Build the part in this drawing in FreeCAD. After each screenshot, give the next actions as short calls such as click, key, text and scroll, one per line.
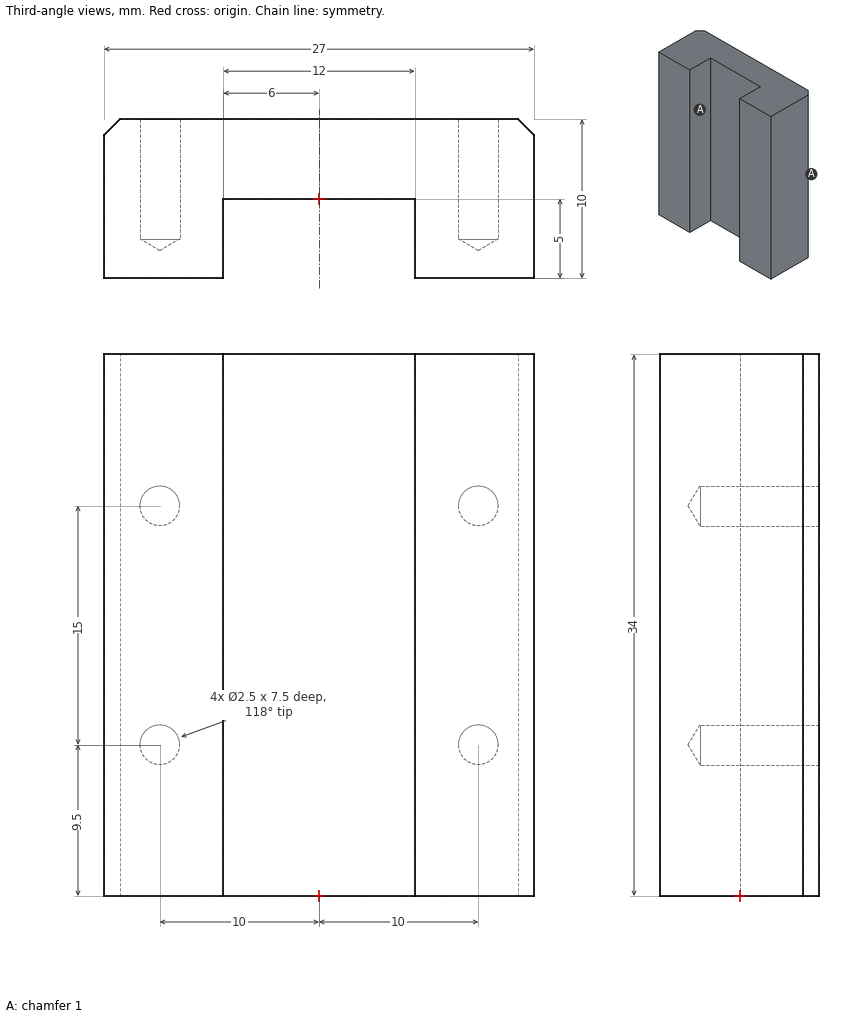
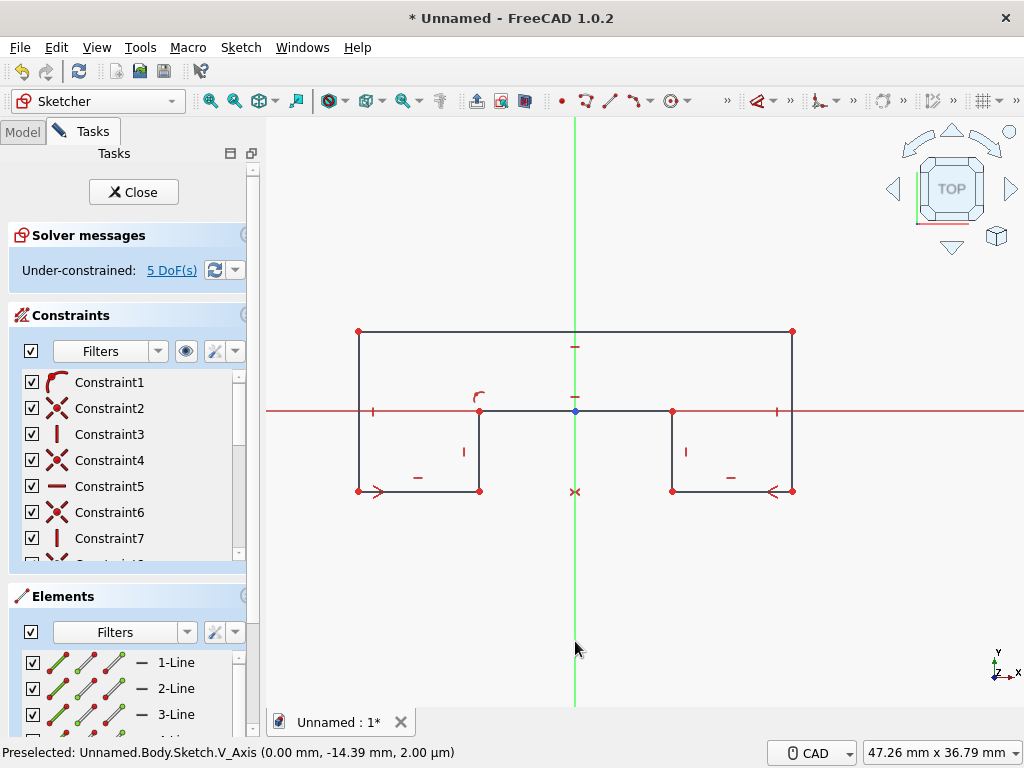
key(d)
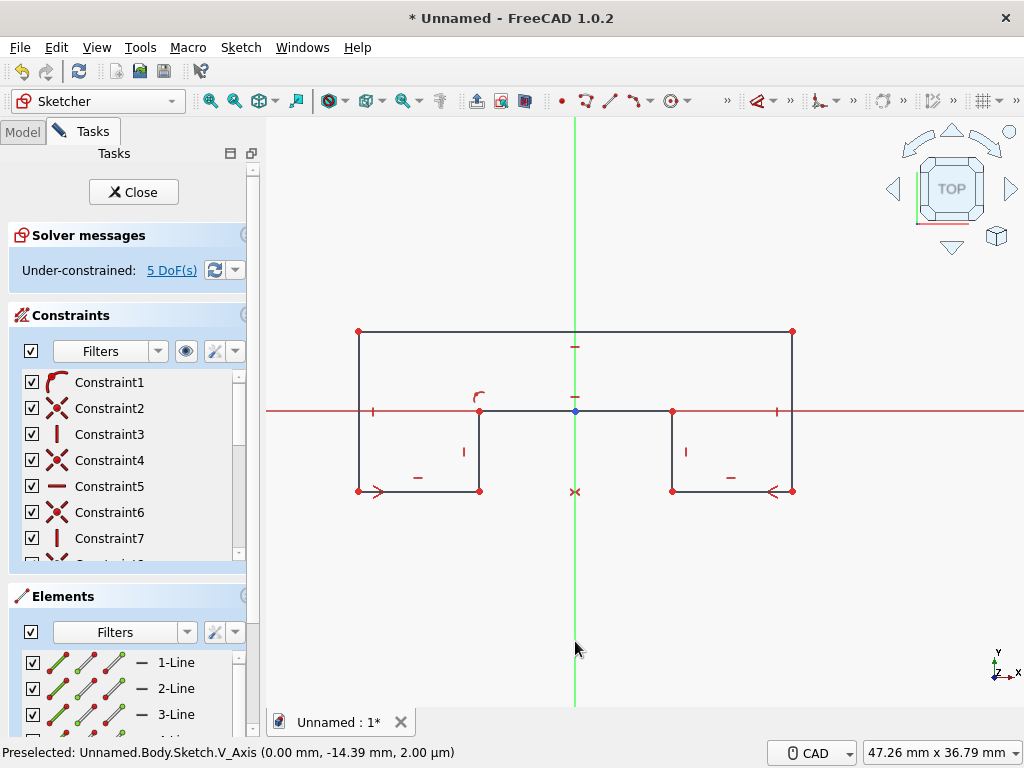
click(672, 435)
click(706, 452)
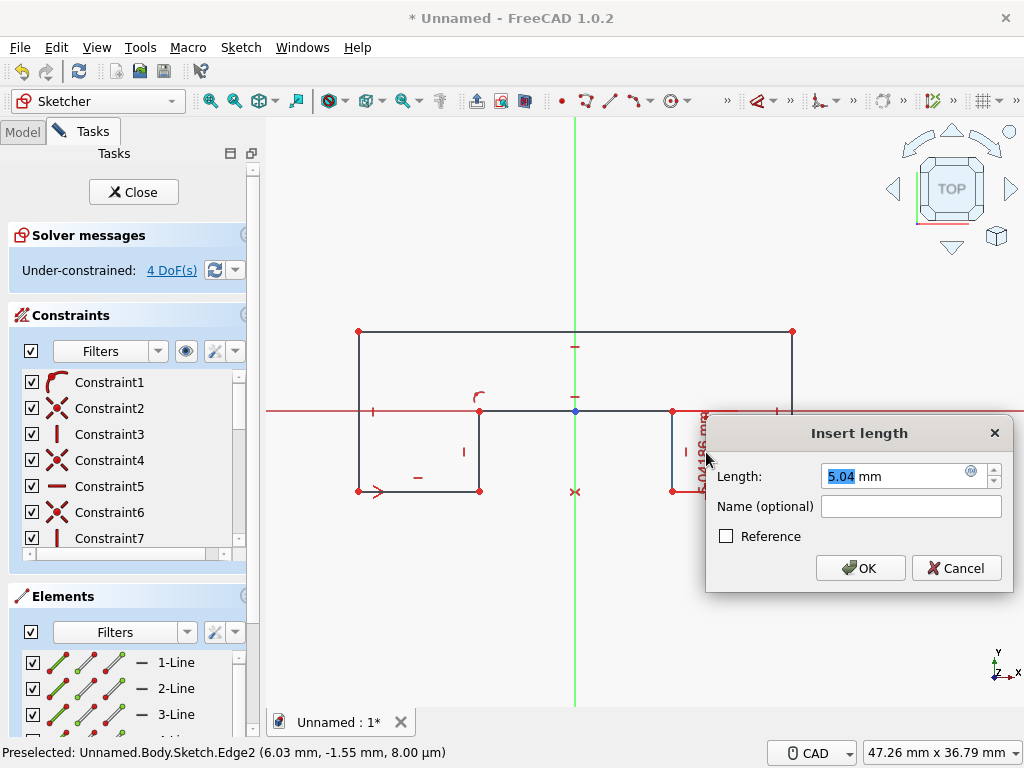
text(5)
key(Return)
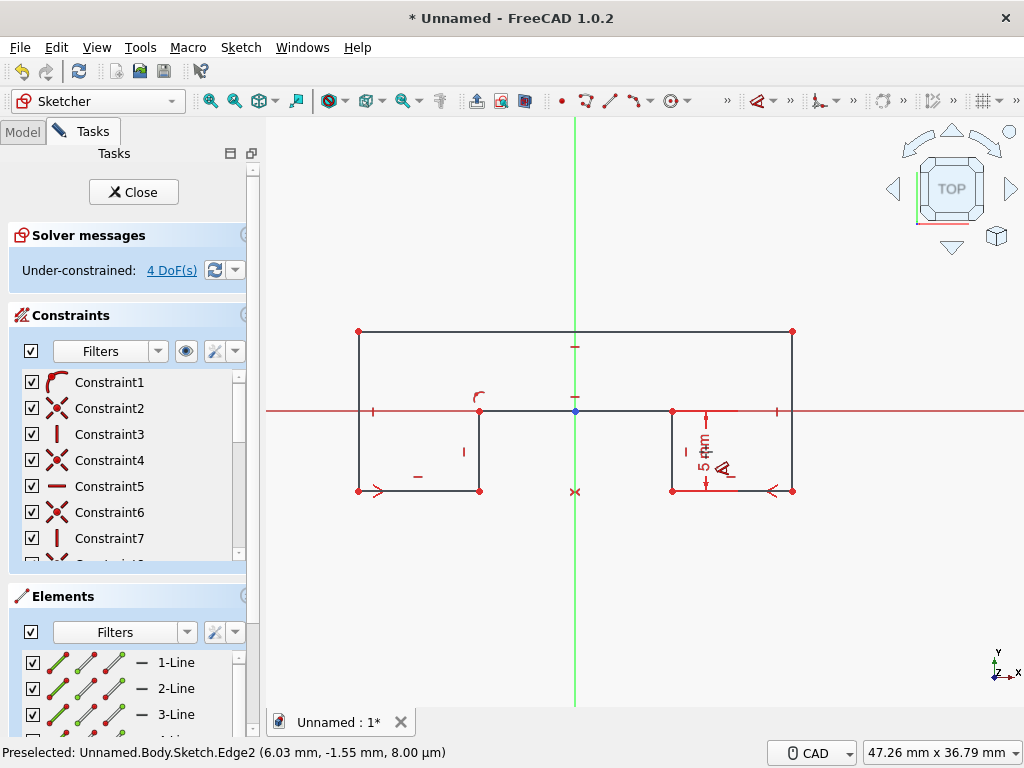
click(537, 411)
click(531, 445)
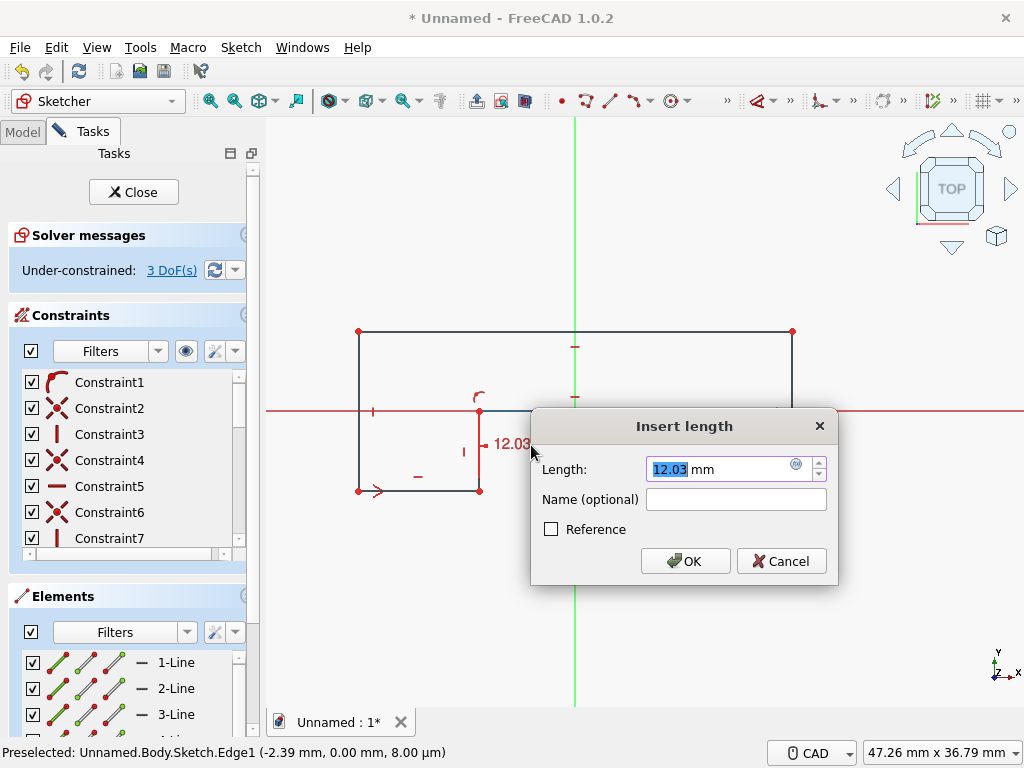
text(12)
key(Return)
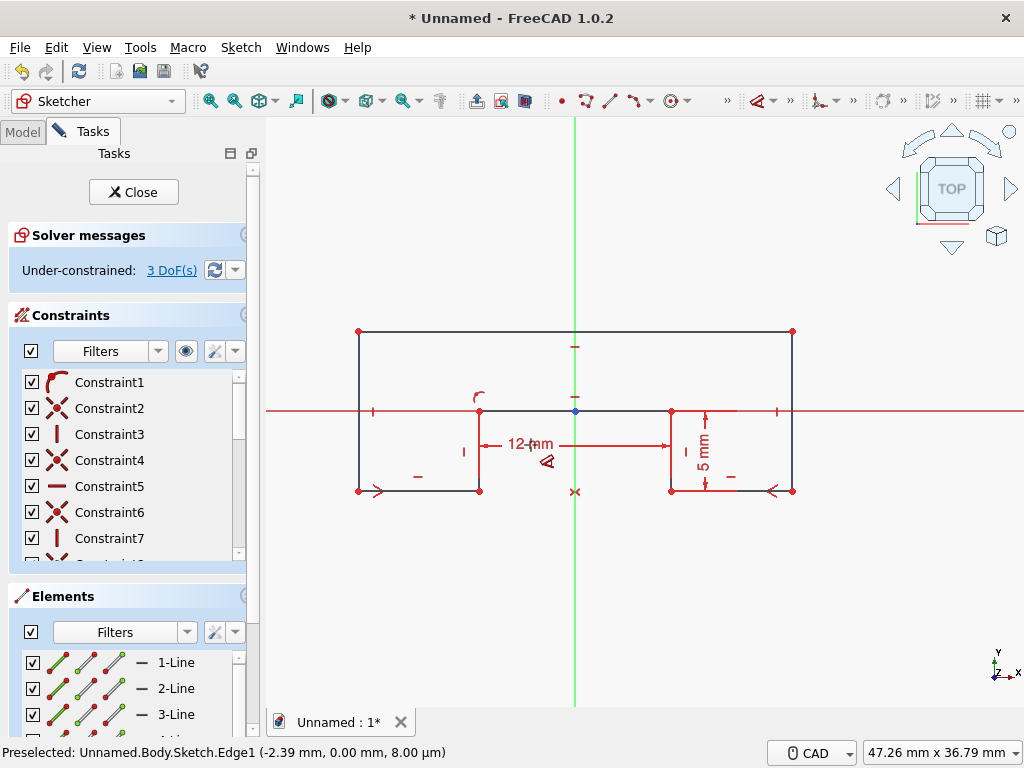
click(792, 444)
click(826, 375)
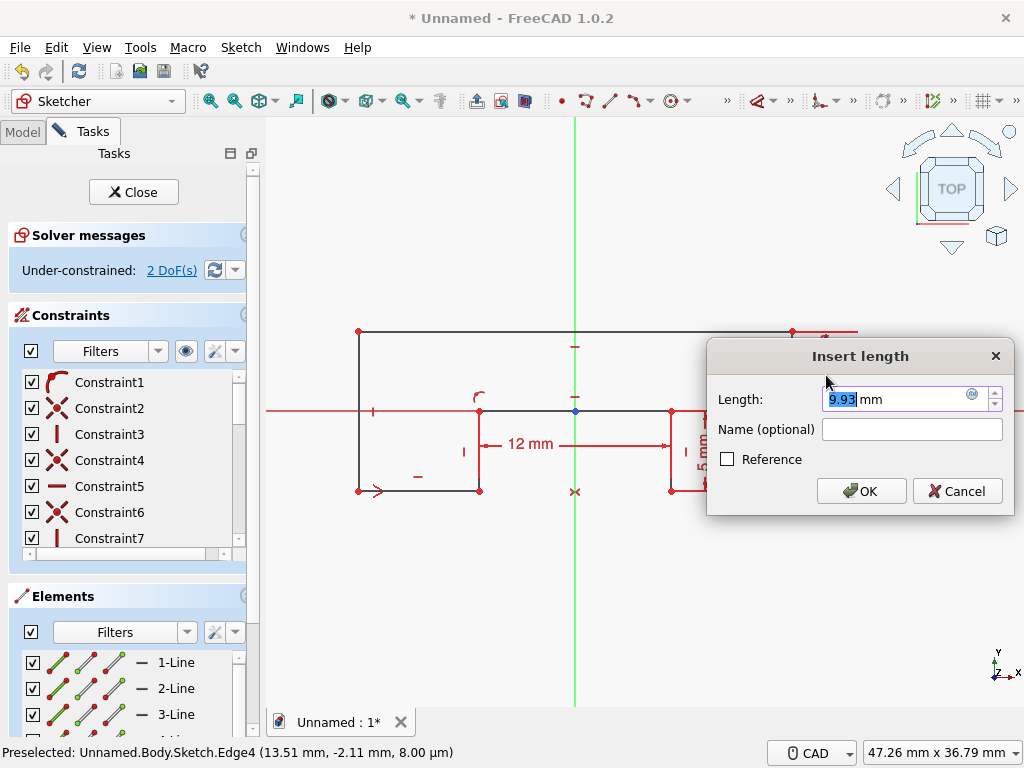
text(10)
key(Return)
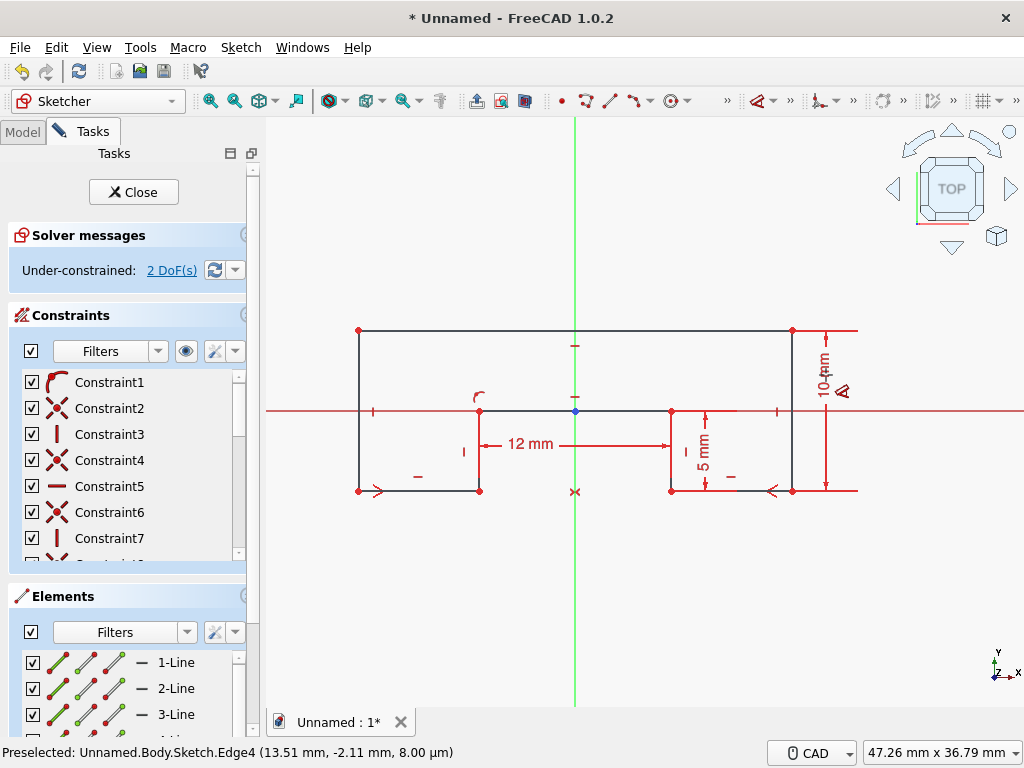
click(662, 331)
click(476, 297)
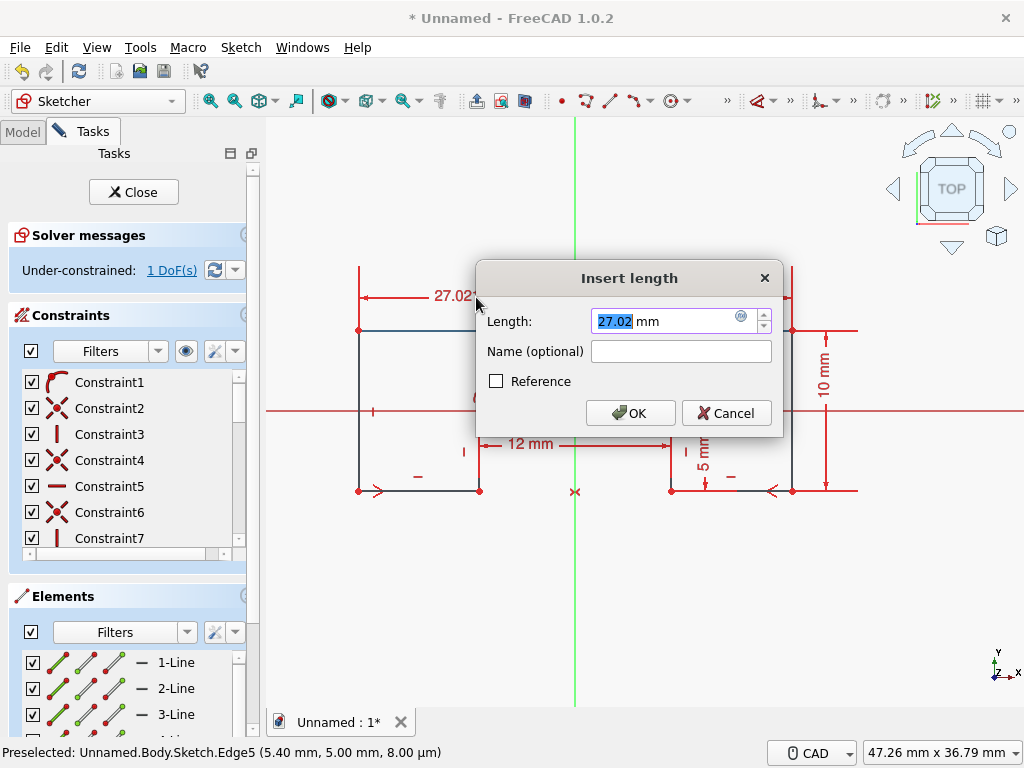
text(27)
key(Return)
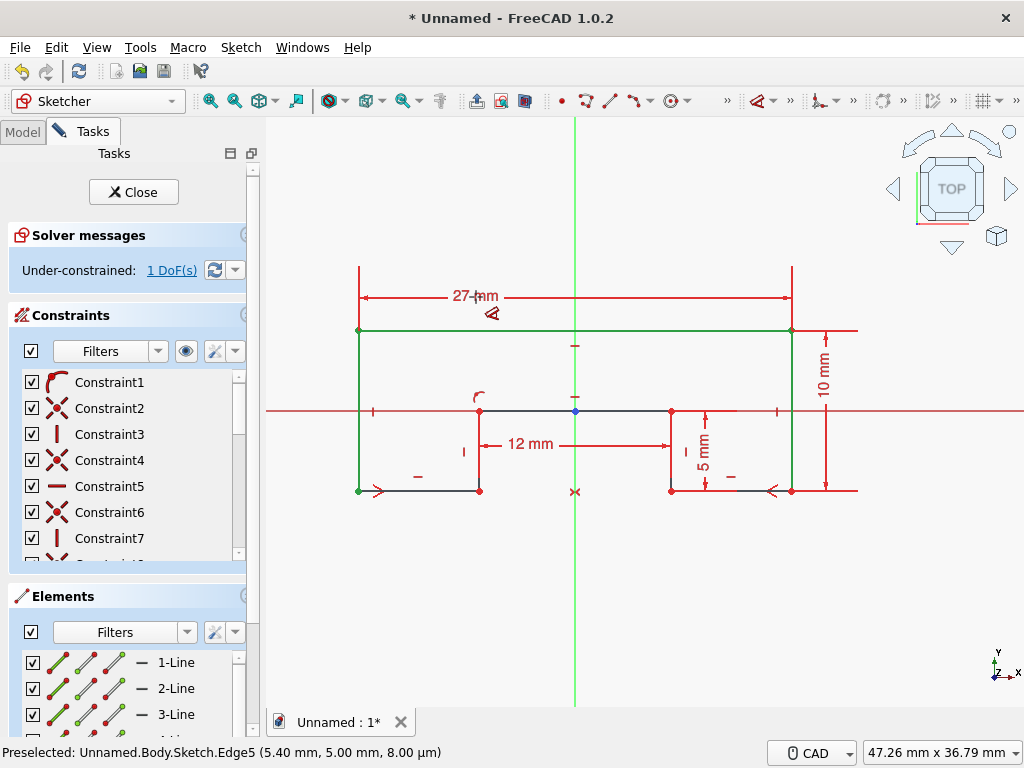
click(479, 411)
click(527, 377)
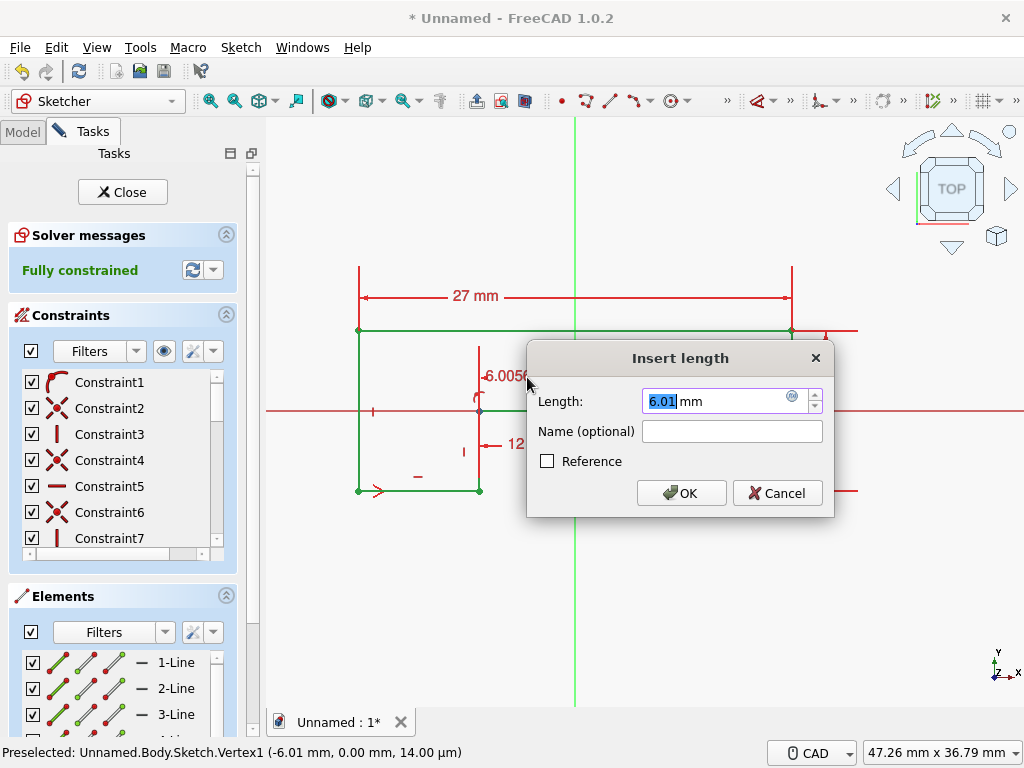
text(6)
key(Return)
key(Escape)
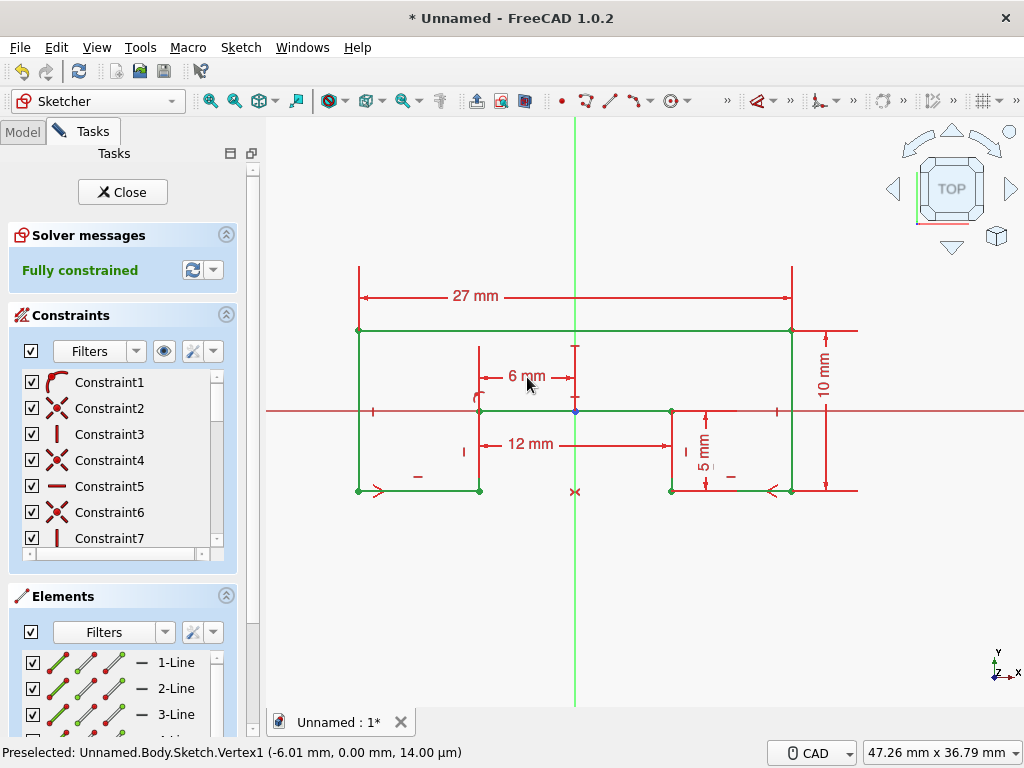
click(123, 192)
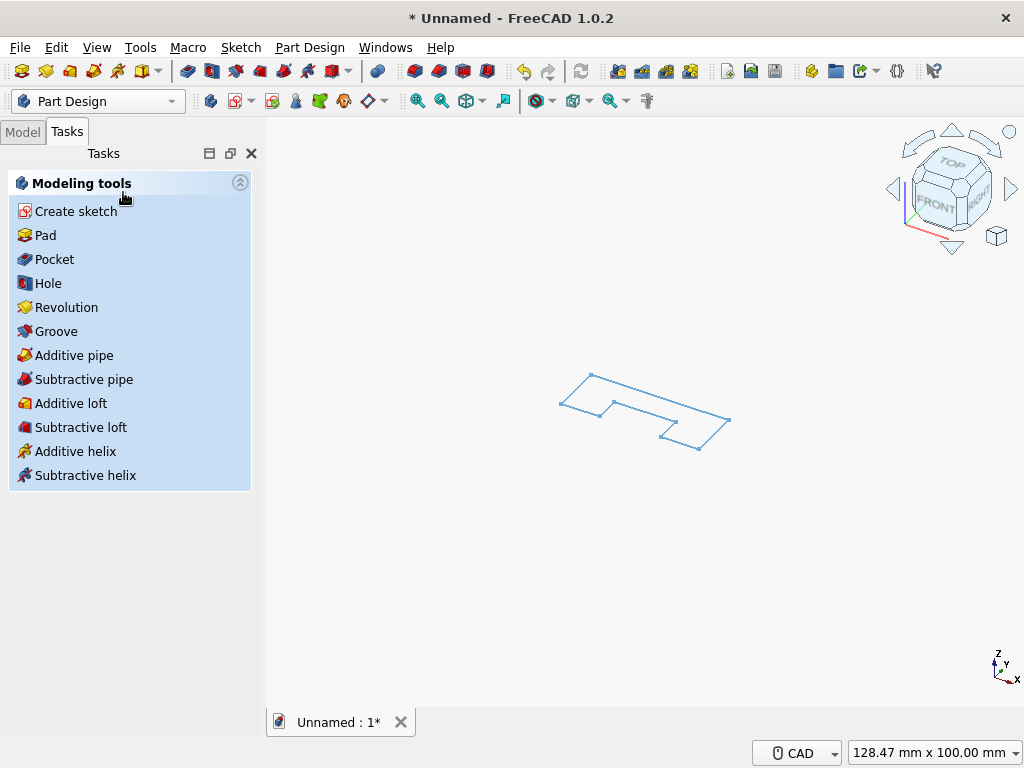
click(22, 72)